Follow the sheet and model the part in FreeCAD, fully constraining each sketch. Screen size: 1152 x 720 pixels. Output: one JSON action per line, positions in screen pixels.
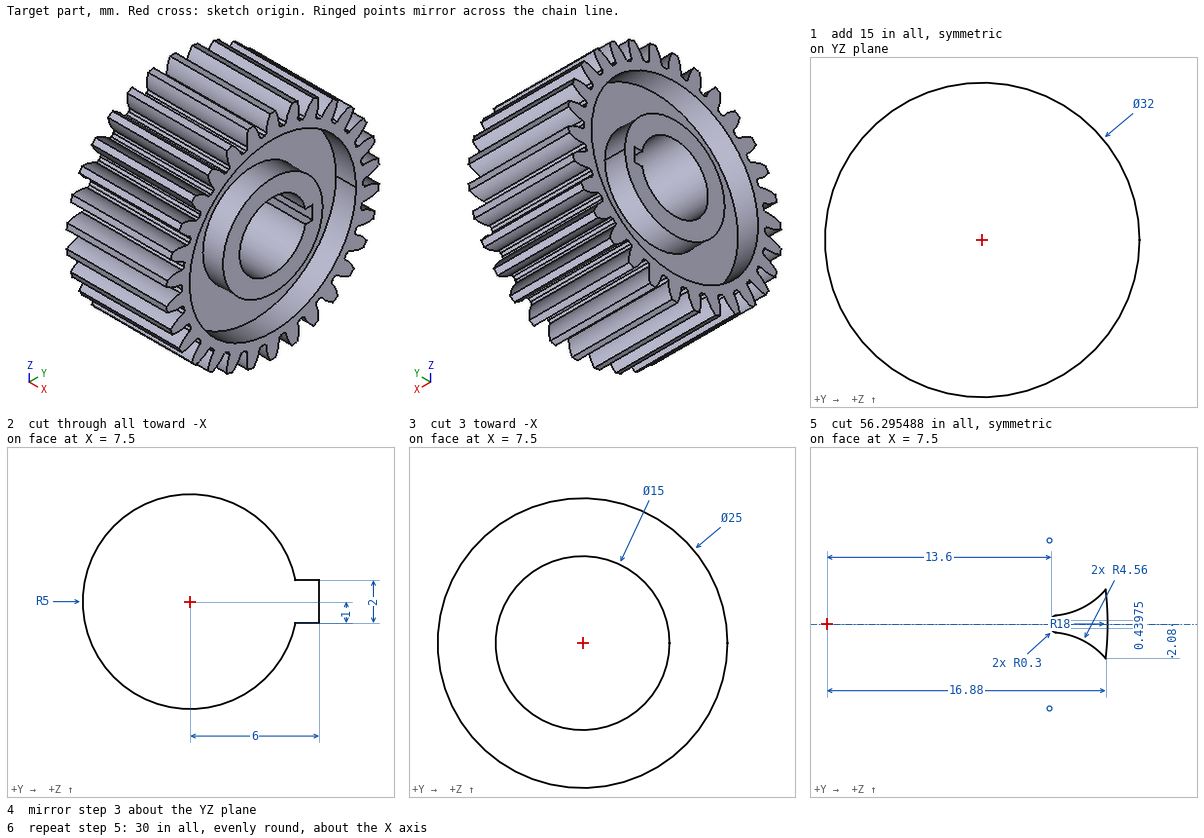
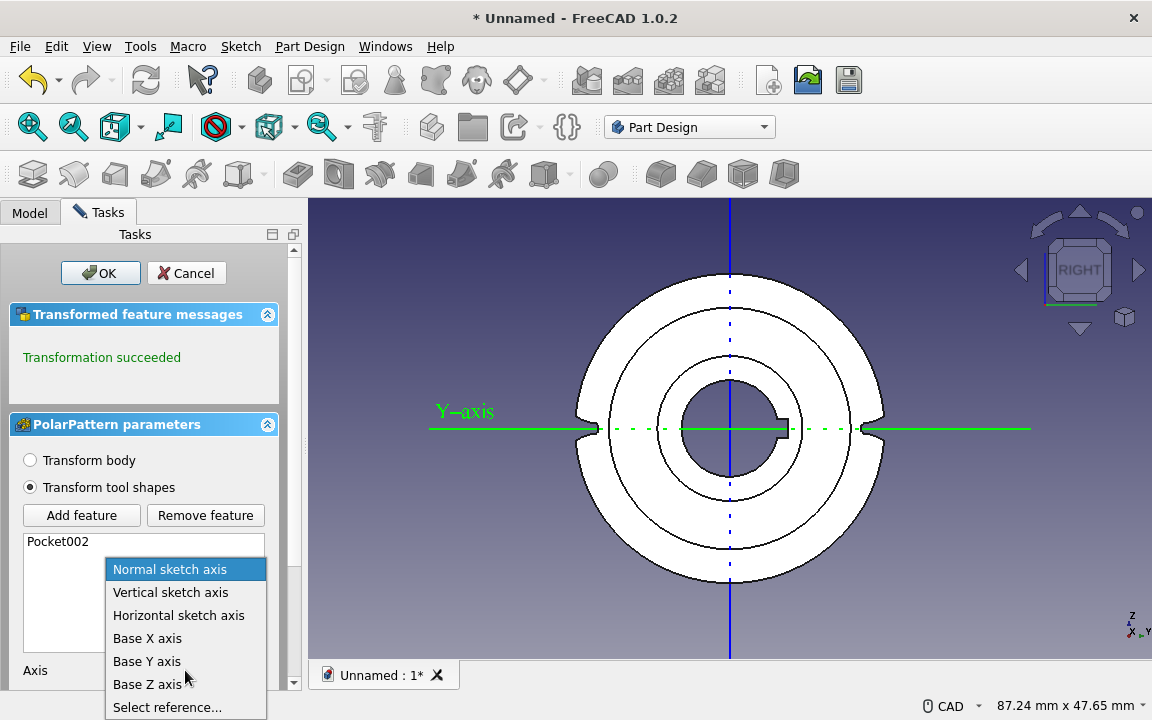
{"action": "left_click", "coordinate": [184, 638]}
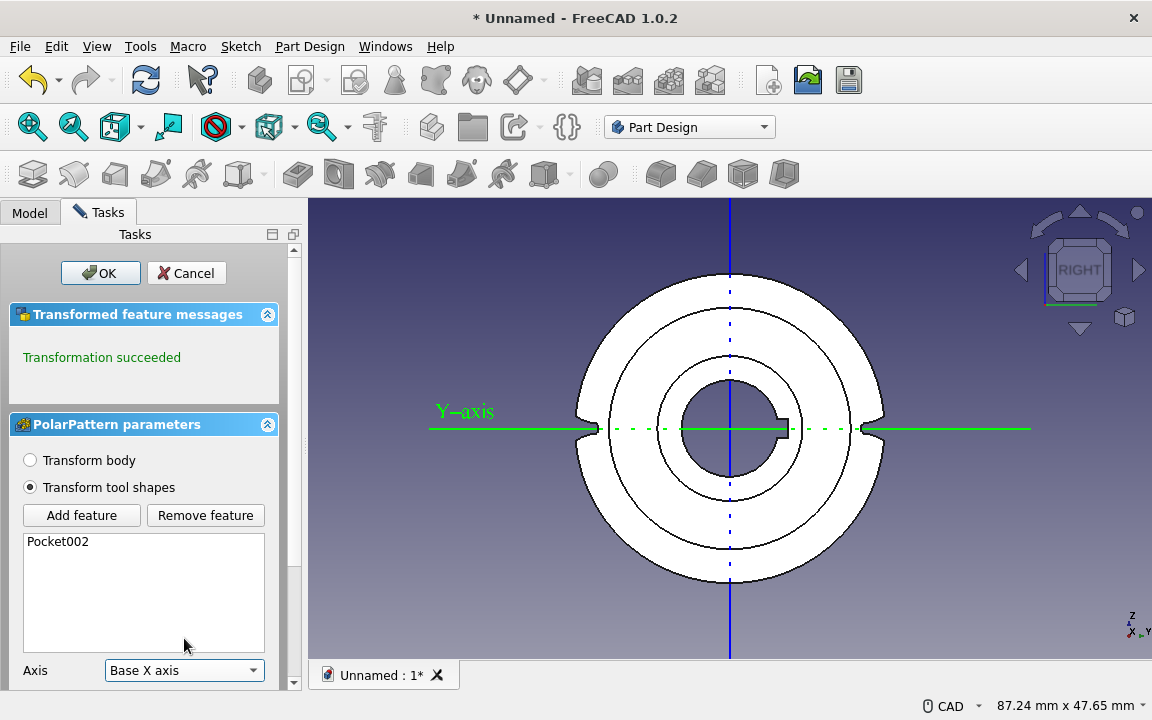
{"action": "scroll", "coordinate": [294, 467], "scroll_direction": "down", "scroll_amount": 3}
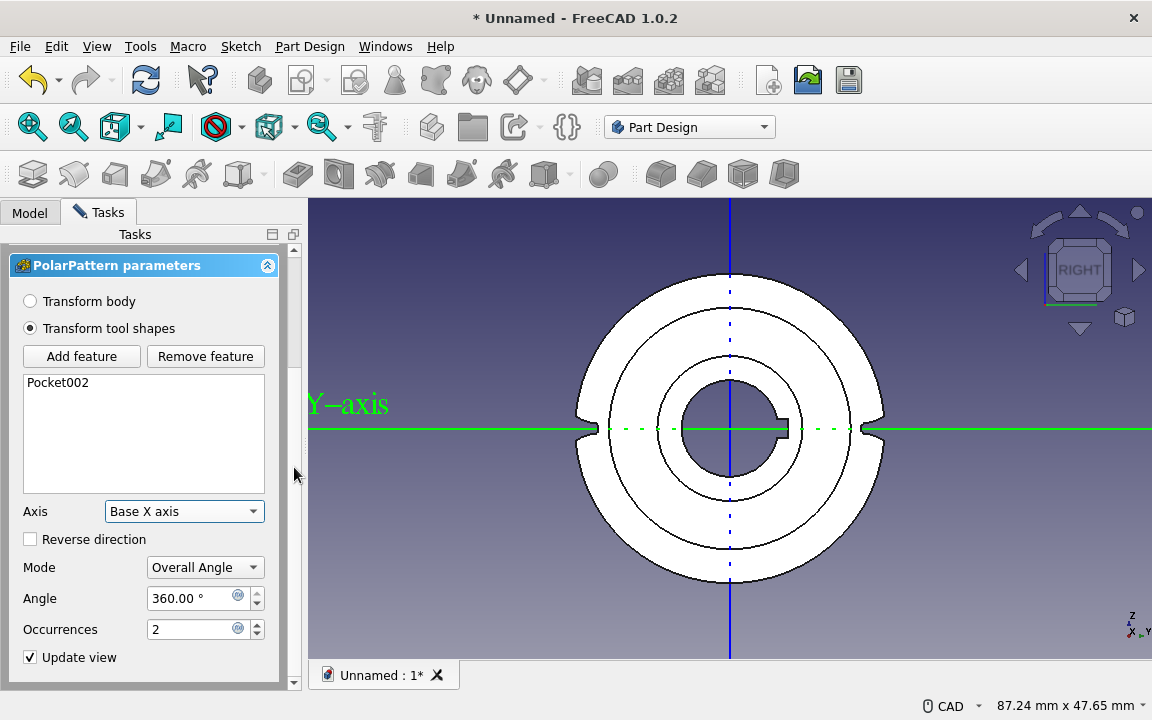
{"action": "triple_click", "coordinate": [199, 630]}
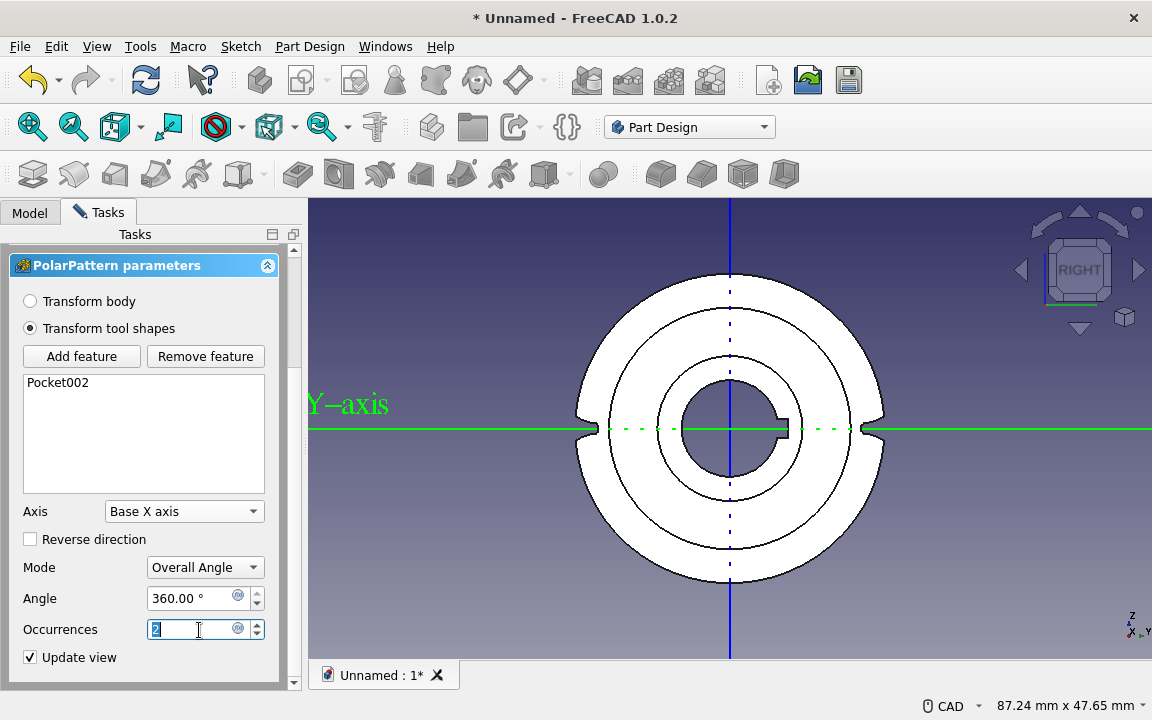
{"action": "type", "text": "30"}
{"action": "key", "text": "Tab"}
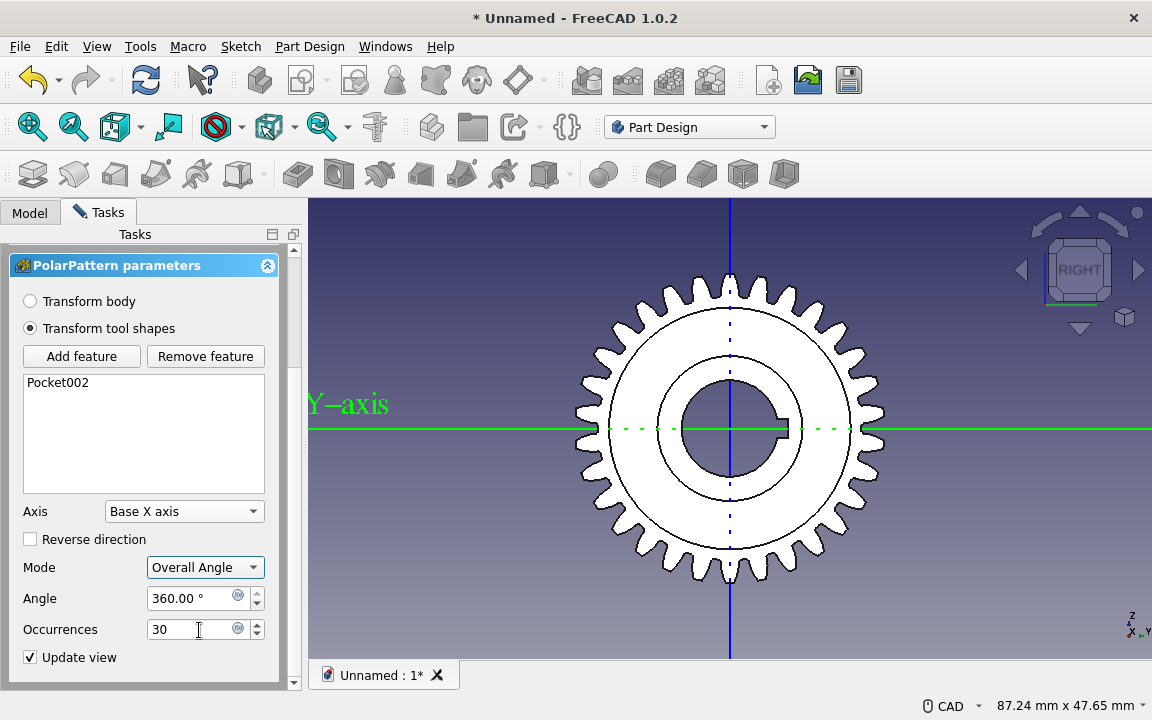
{"action": "scroll", "coordinate": [294, 467], "scroll_direction": "up", "scroll_amount": 4}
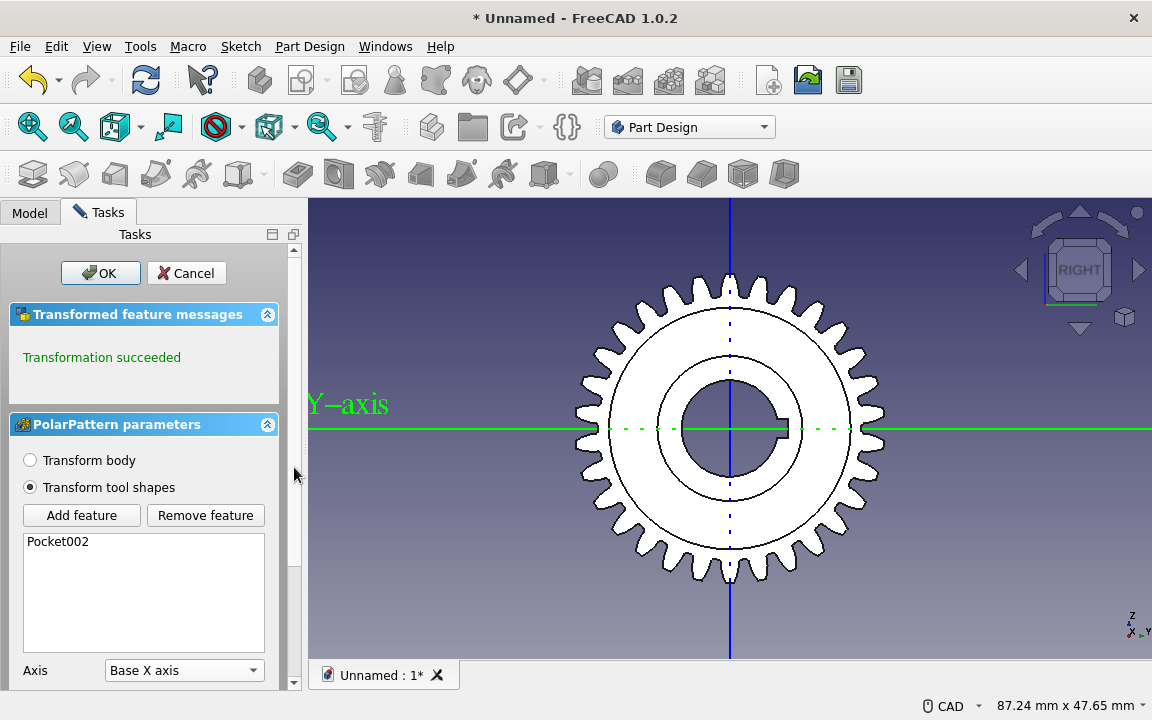
{"action": "left_click", "coordinate": [101, 273]}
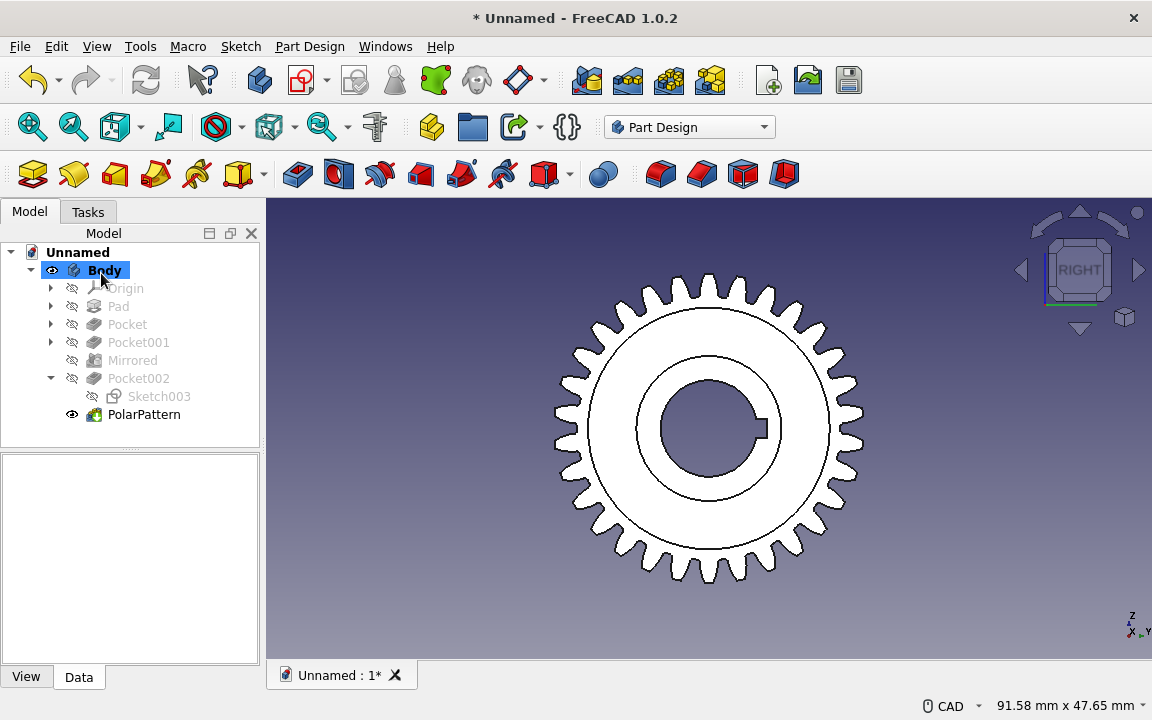
{"action": "key", "text": "0"}